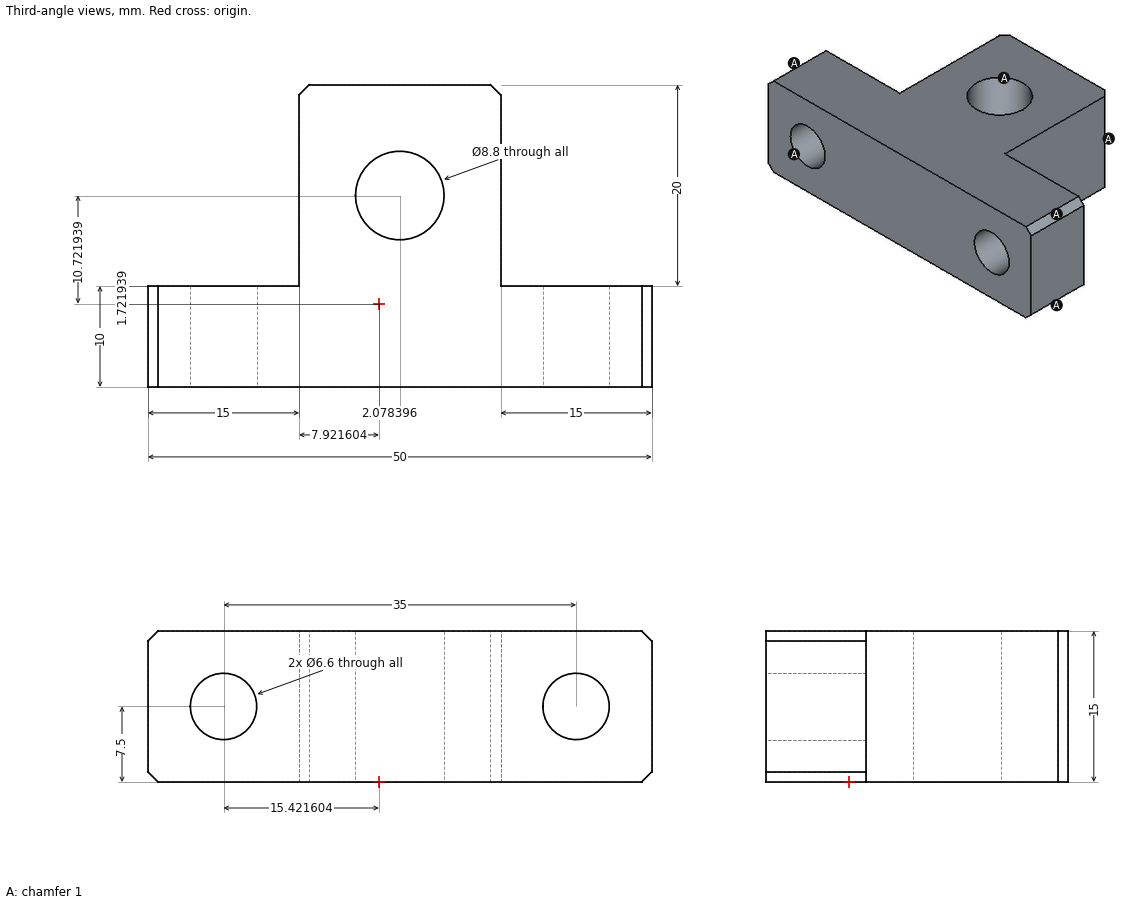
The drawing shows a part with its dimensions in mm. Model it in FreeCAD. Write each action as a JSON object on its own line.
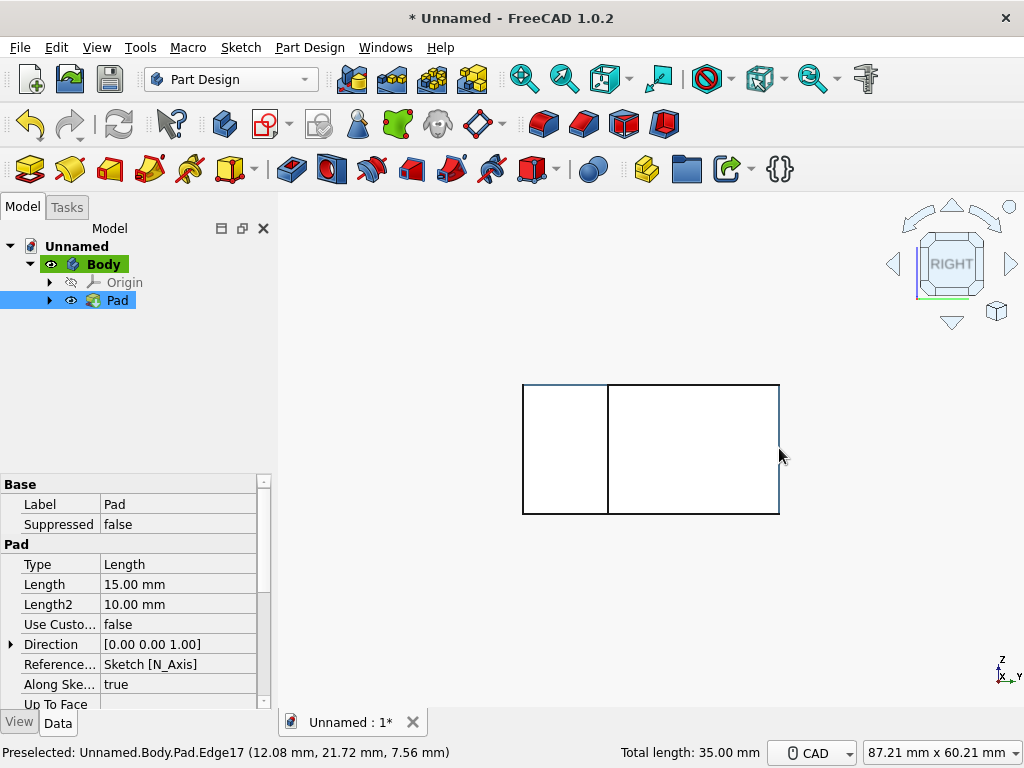
{"action": "left_click", "coordinate": [565, 513], "text": "ctrl"}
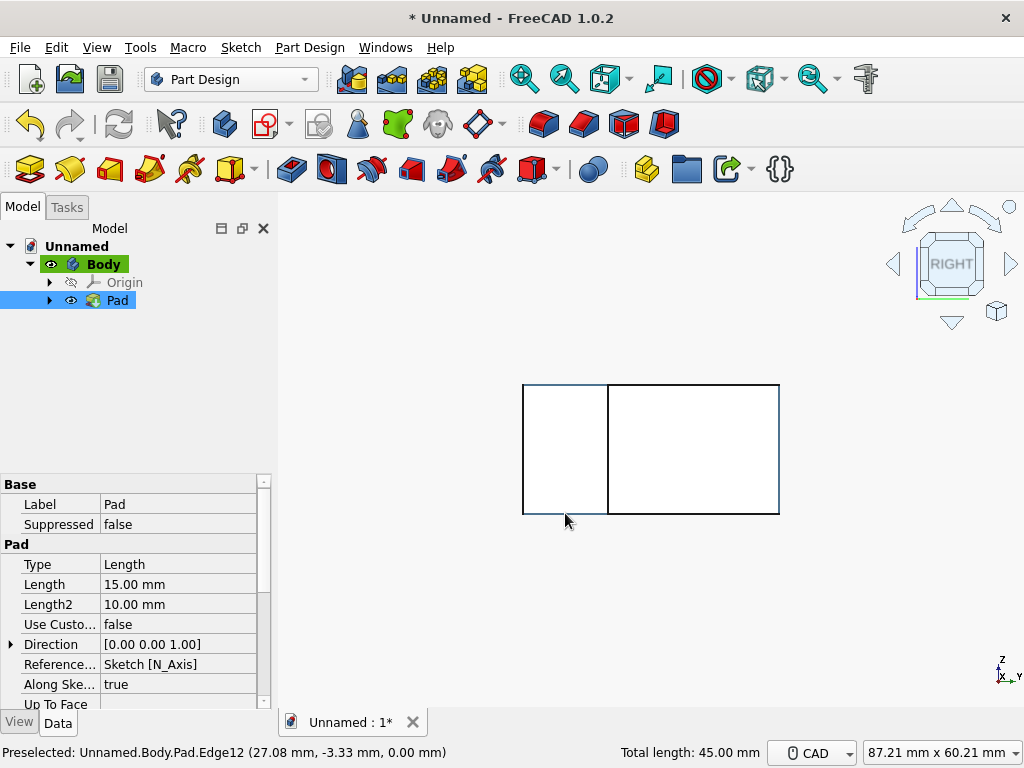
{"action": "key", "text": "5"}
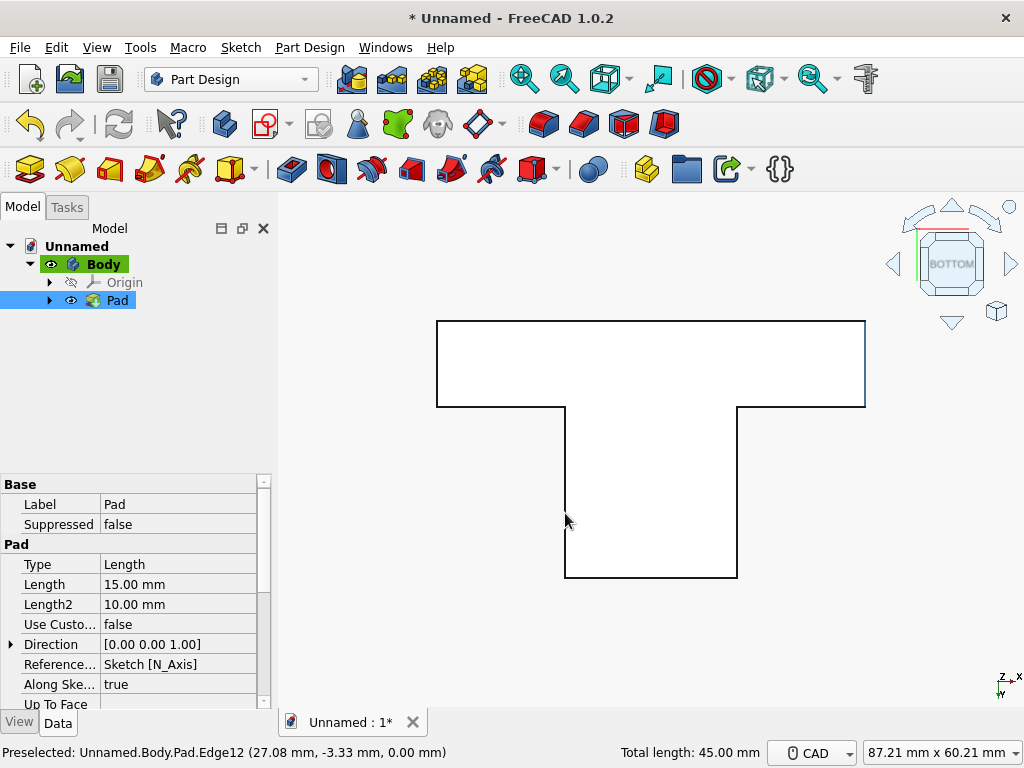
{"action": "left_click", "coordinate": [437, 363], "text": "ctrl"}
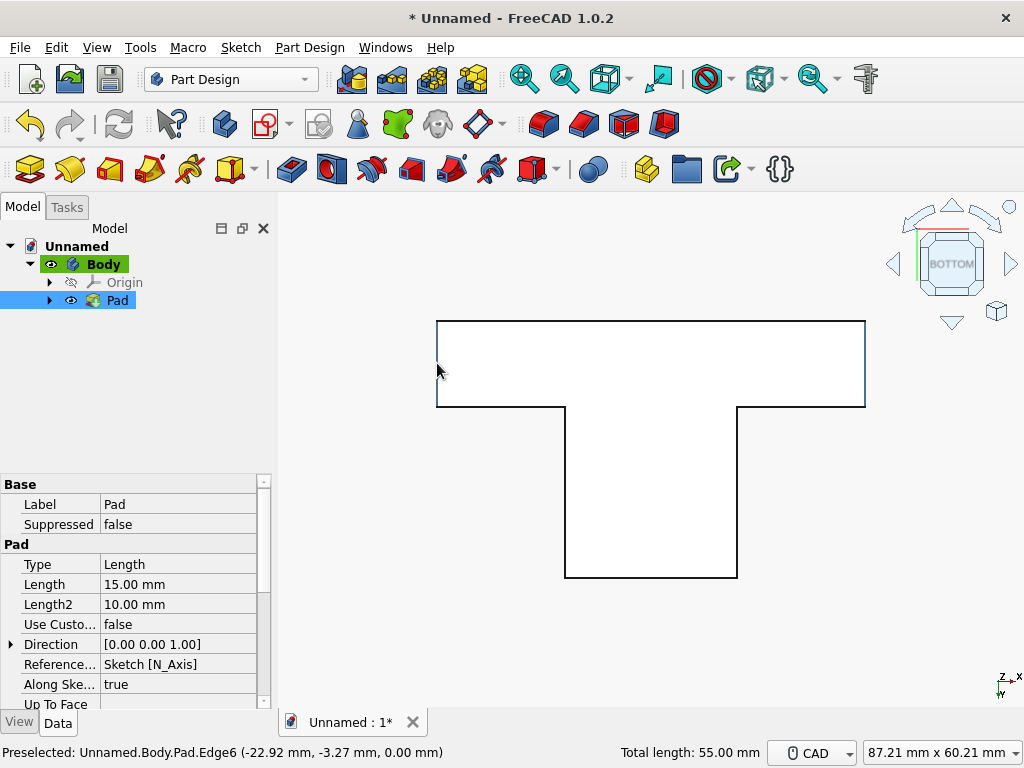
{"action": "key", "text": "4"}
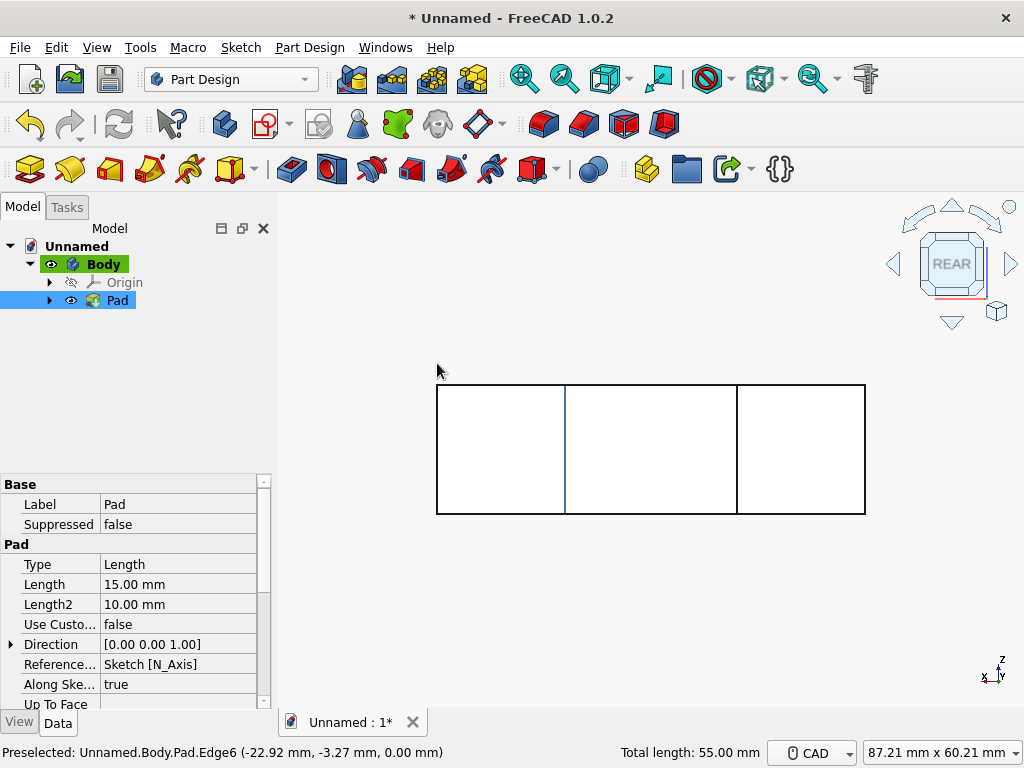
{"action": "left_click", "coordinate": [737, 448], "text": "ctrl"}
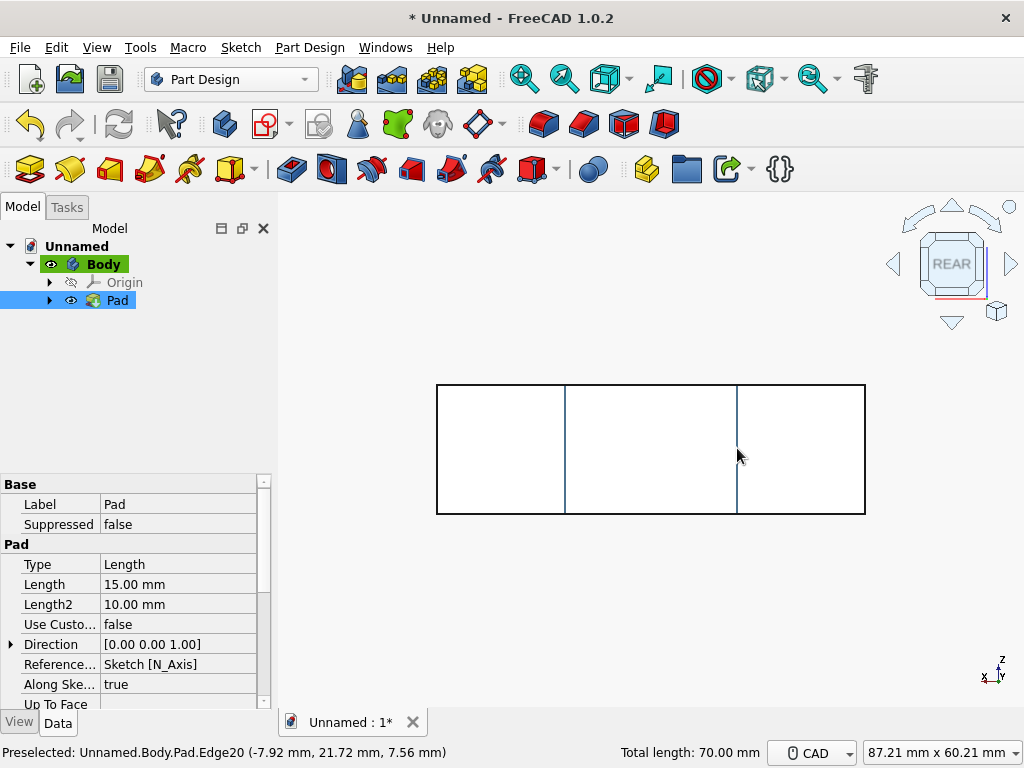
{"action": "left_click", "coordinate": [584, 124]}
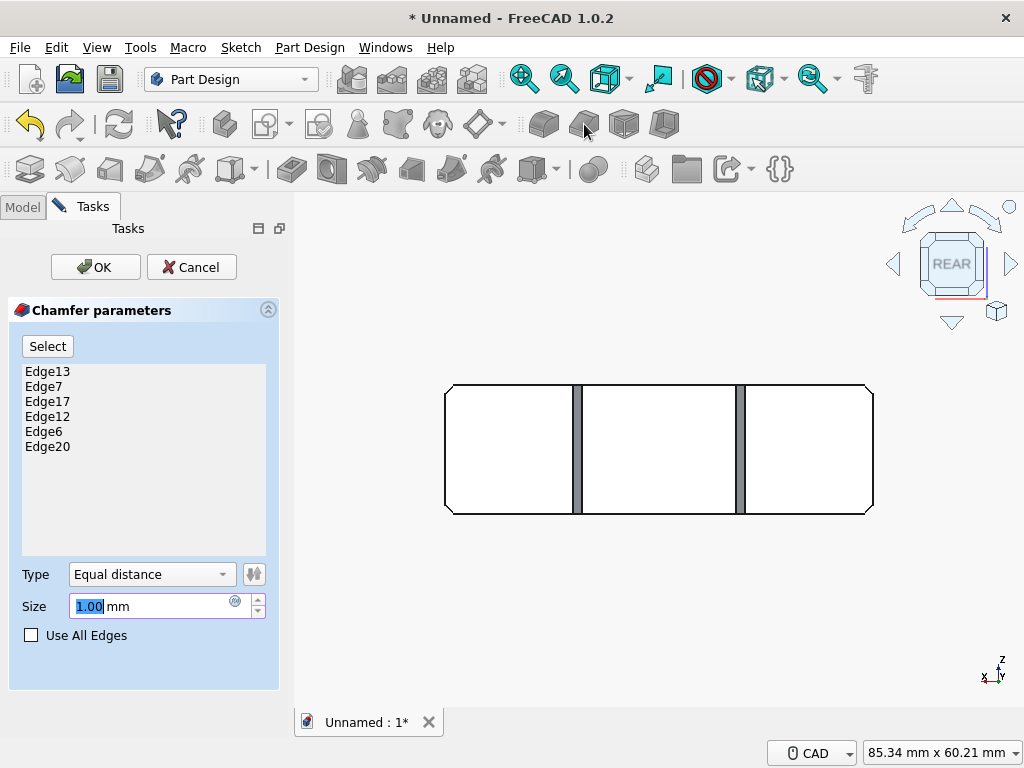
{"action": "type", "text": "1"}
{"action": "key", "text": "Tab"}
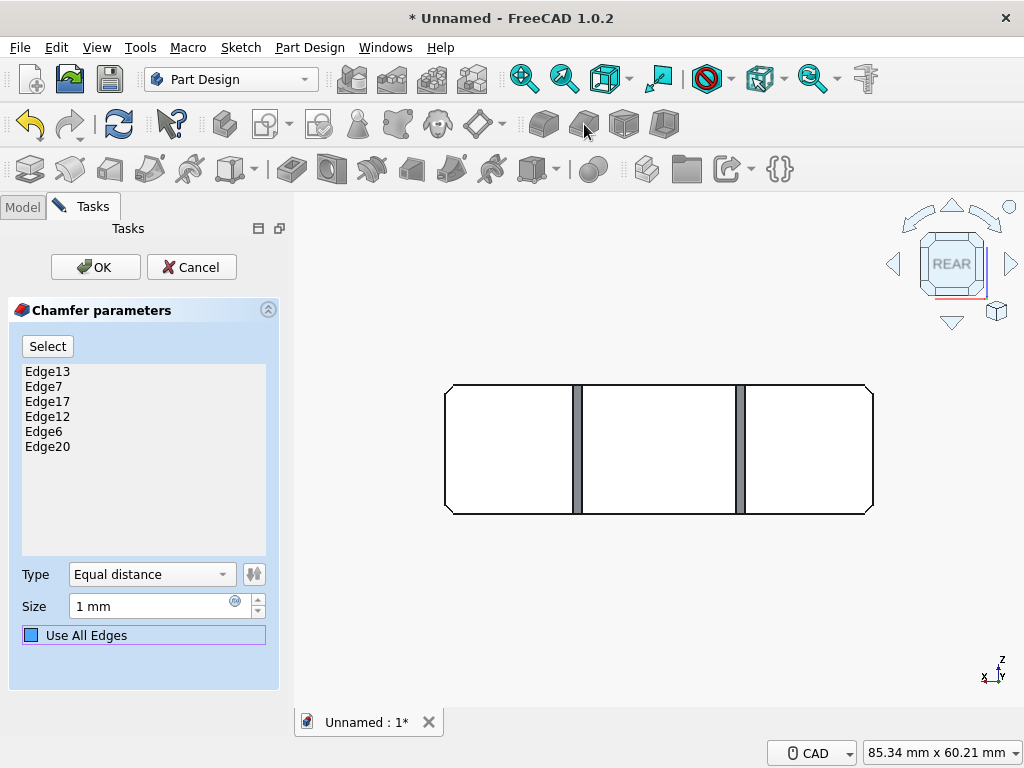
{"action": "left_click", "coordinate": [96, 267]}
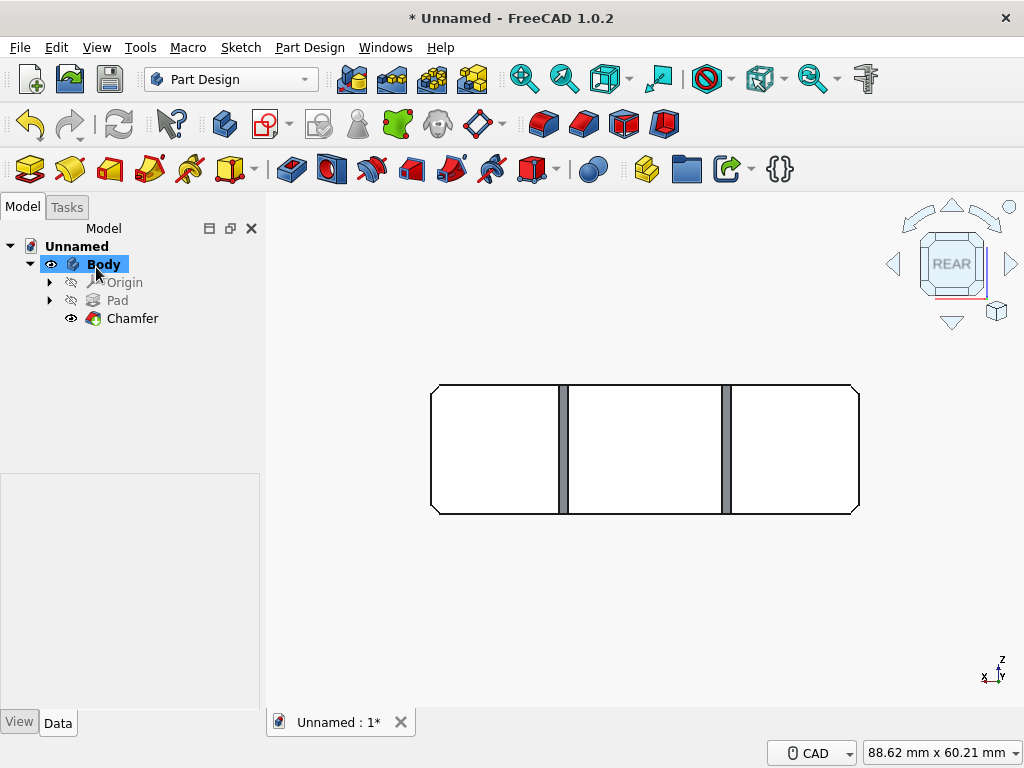
{"action": "left_click", "coordinate": [795, 448]}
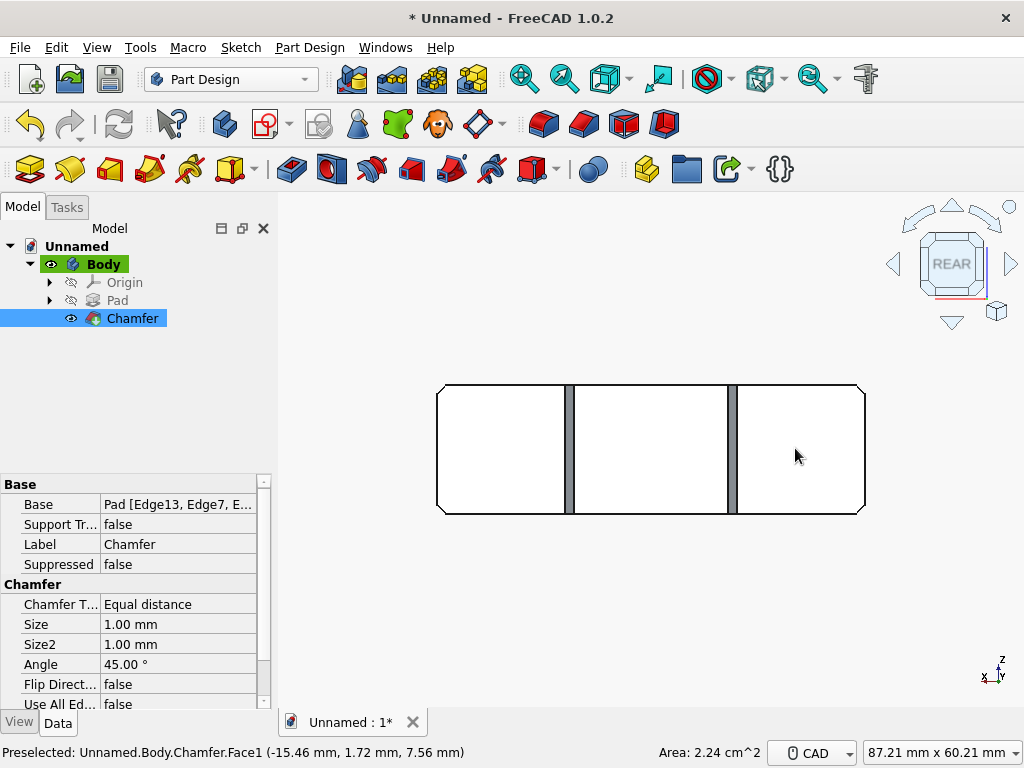
{"action": "left_click", "coordinate": [266, 124]}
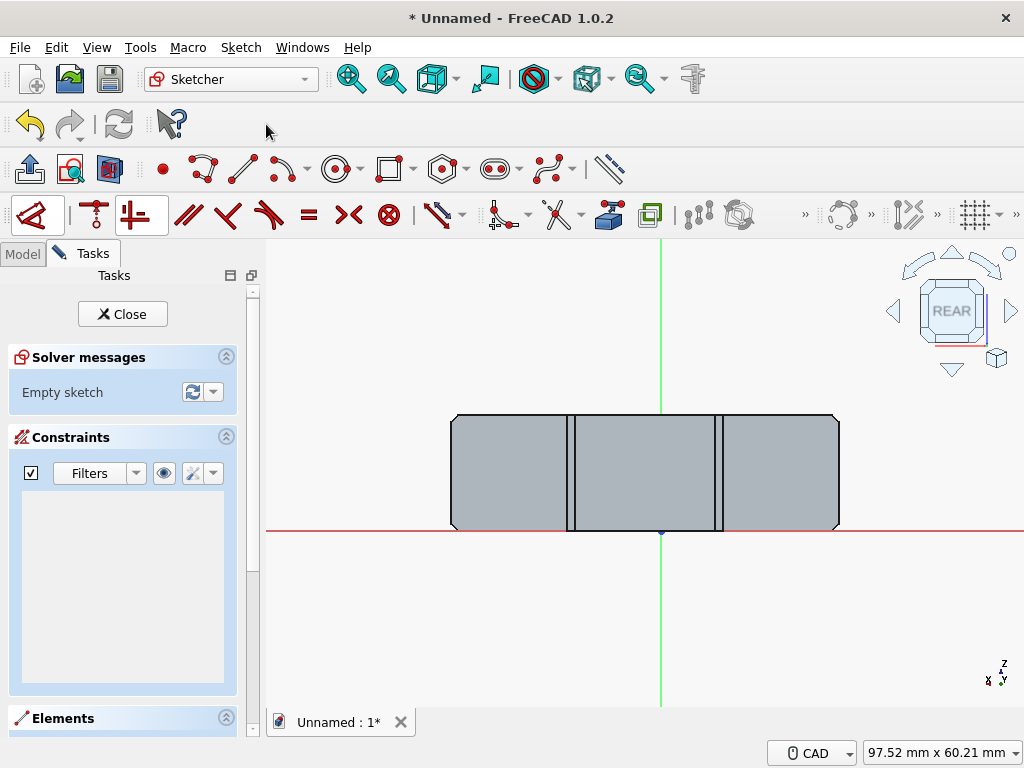
{"action": "left_click", "coordinate": [110, 170]}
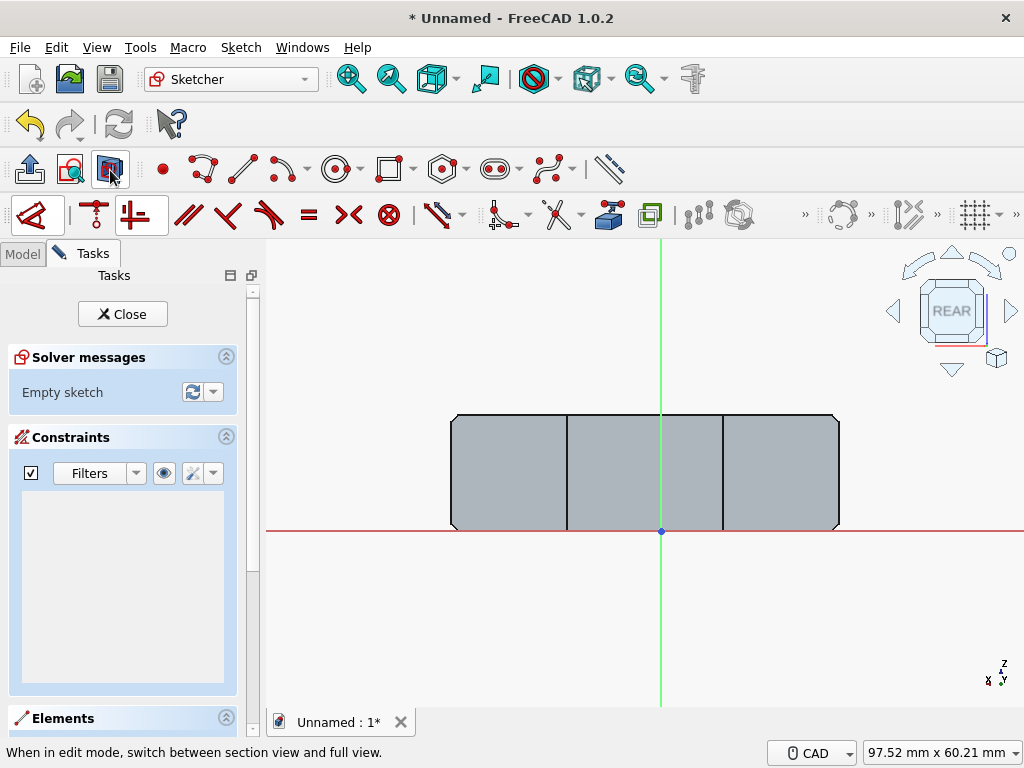
{"action": "left_click", "coordinate": [336, 170]}